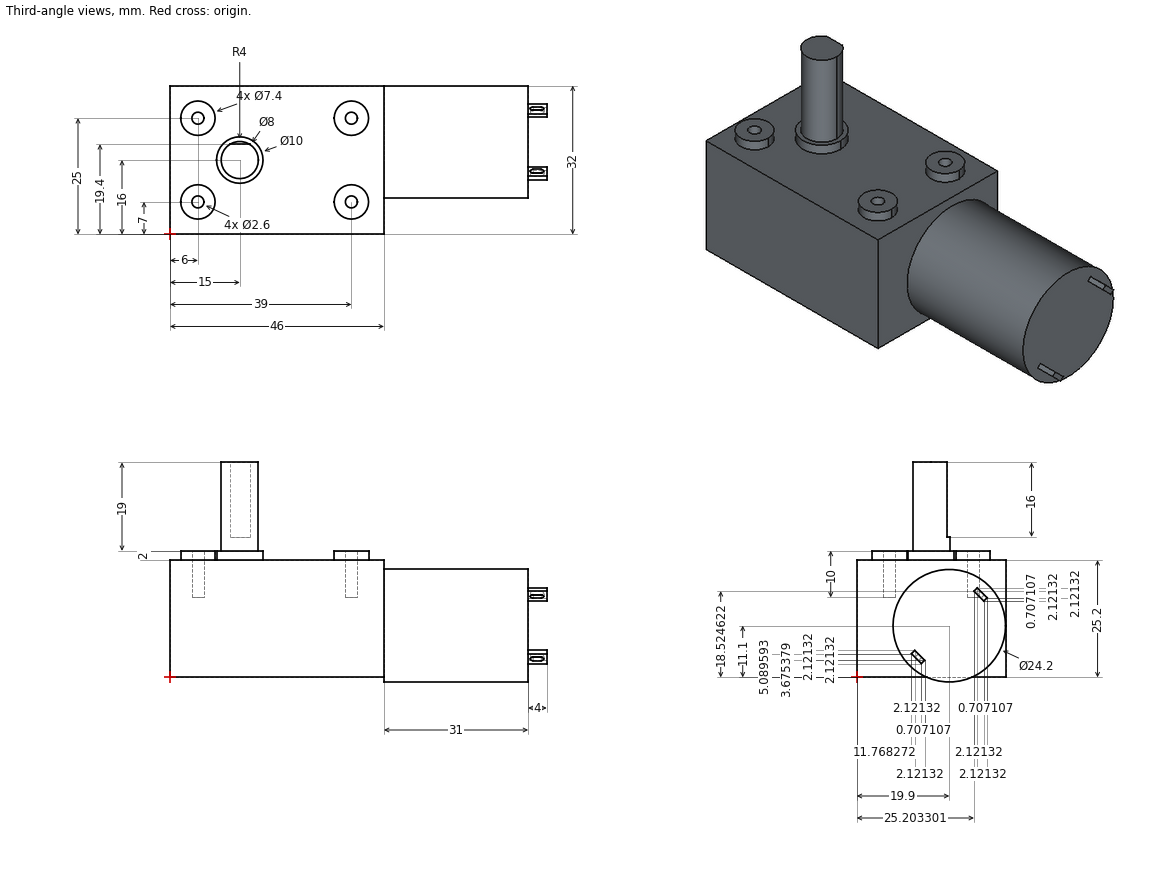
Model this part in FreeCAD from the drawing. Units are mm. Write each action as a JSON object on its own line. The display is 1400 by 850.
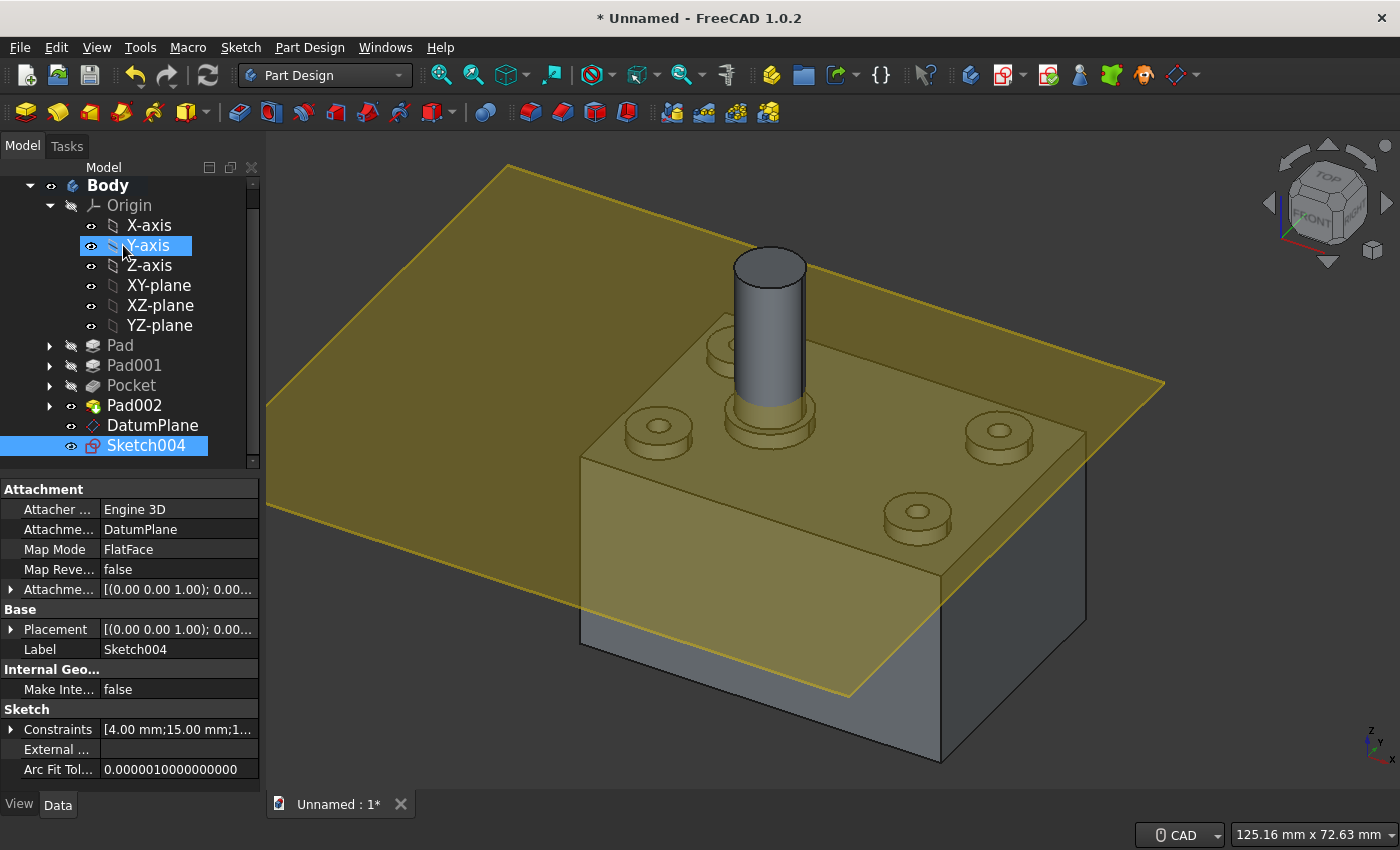
{"action": "left_click", "coordinate": [240, 112]}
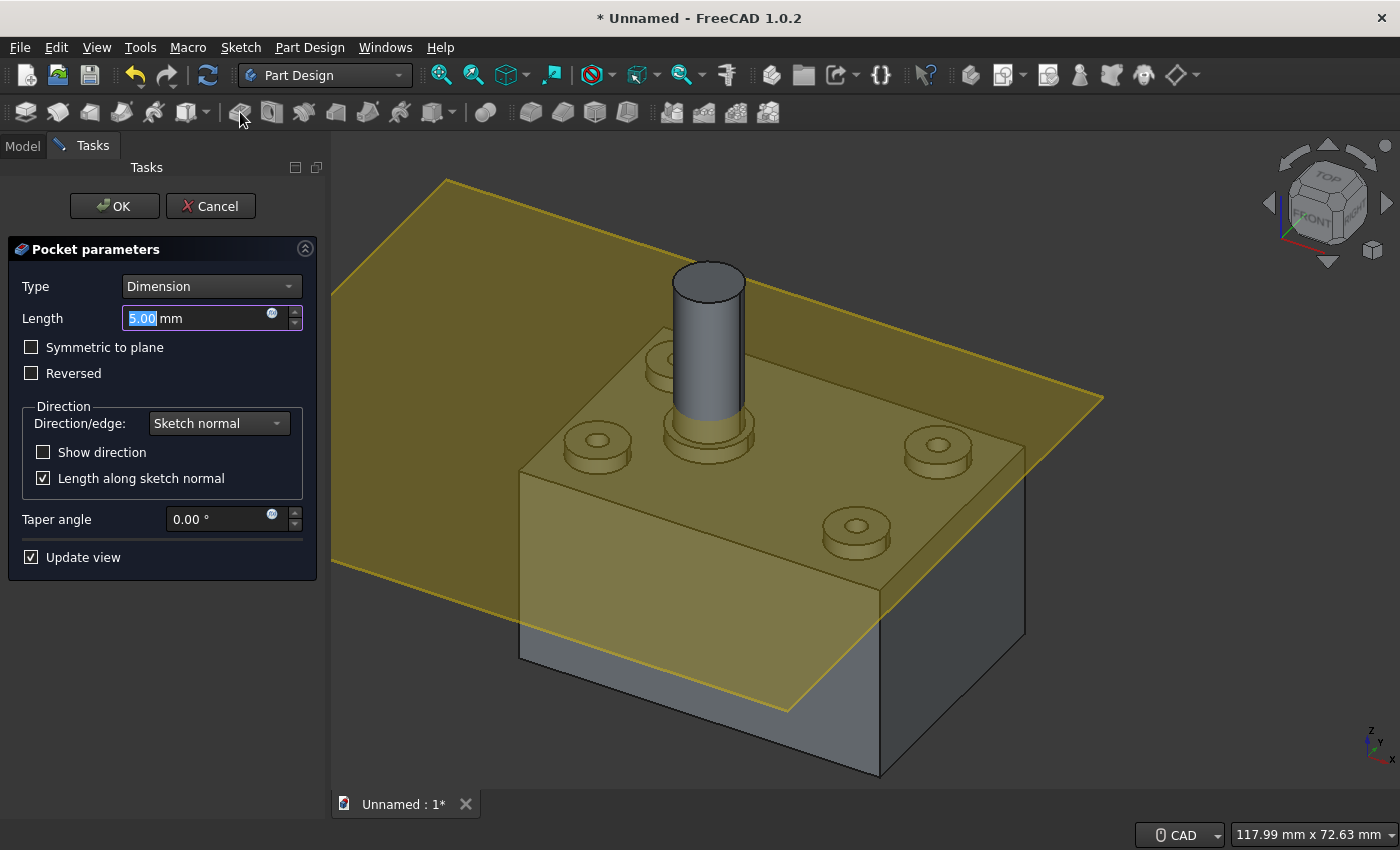
{"action": "type", "text": "16"}
{"action": "key", "text": "Tab"}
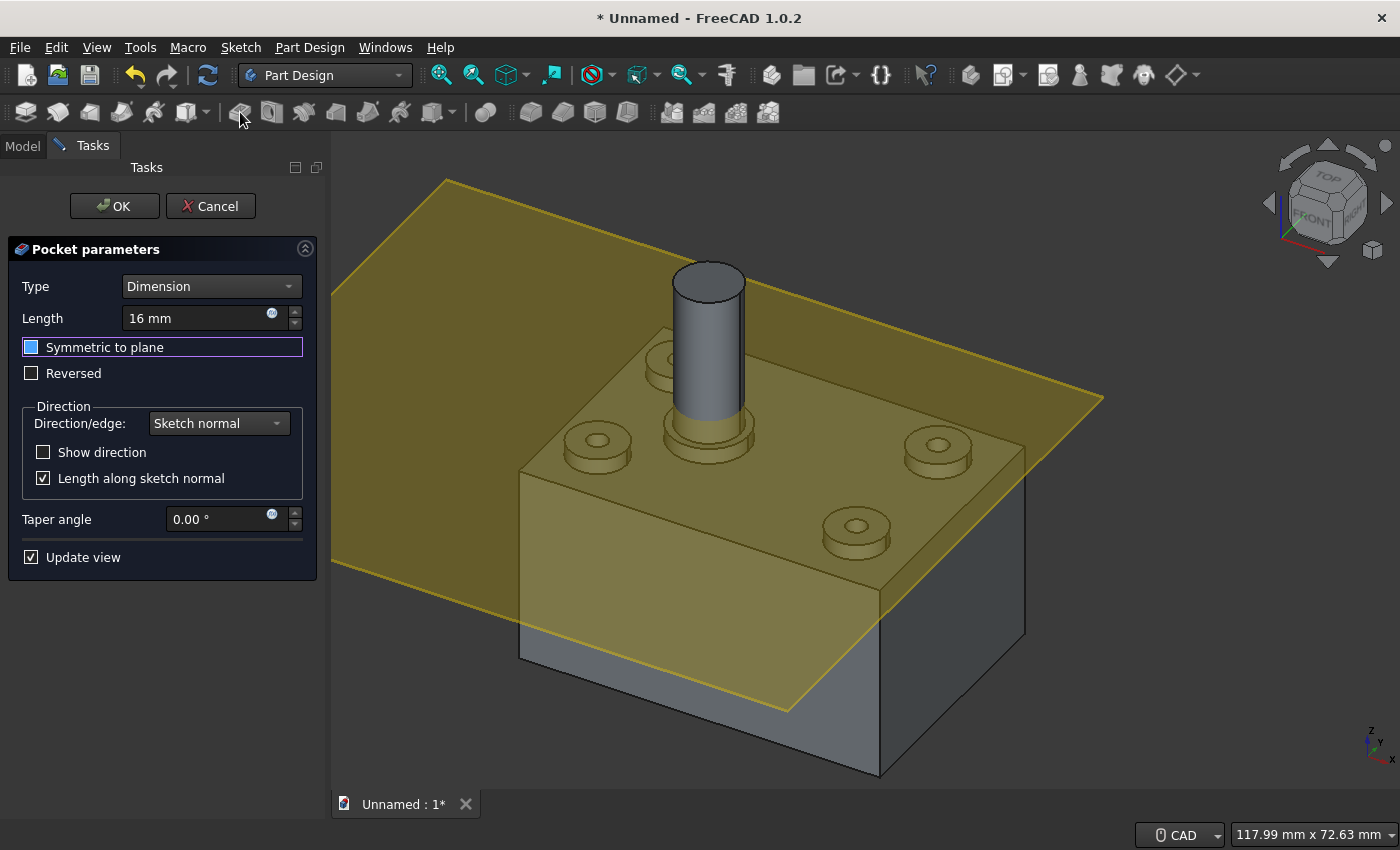
{"action": "left_click", "coordinate": [30, 373]}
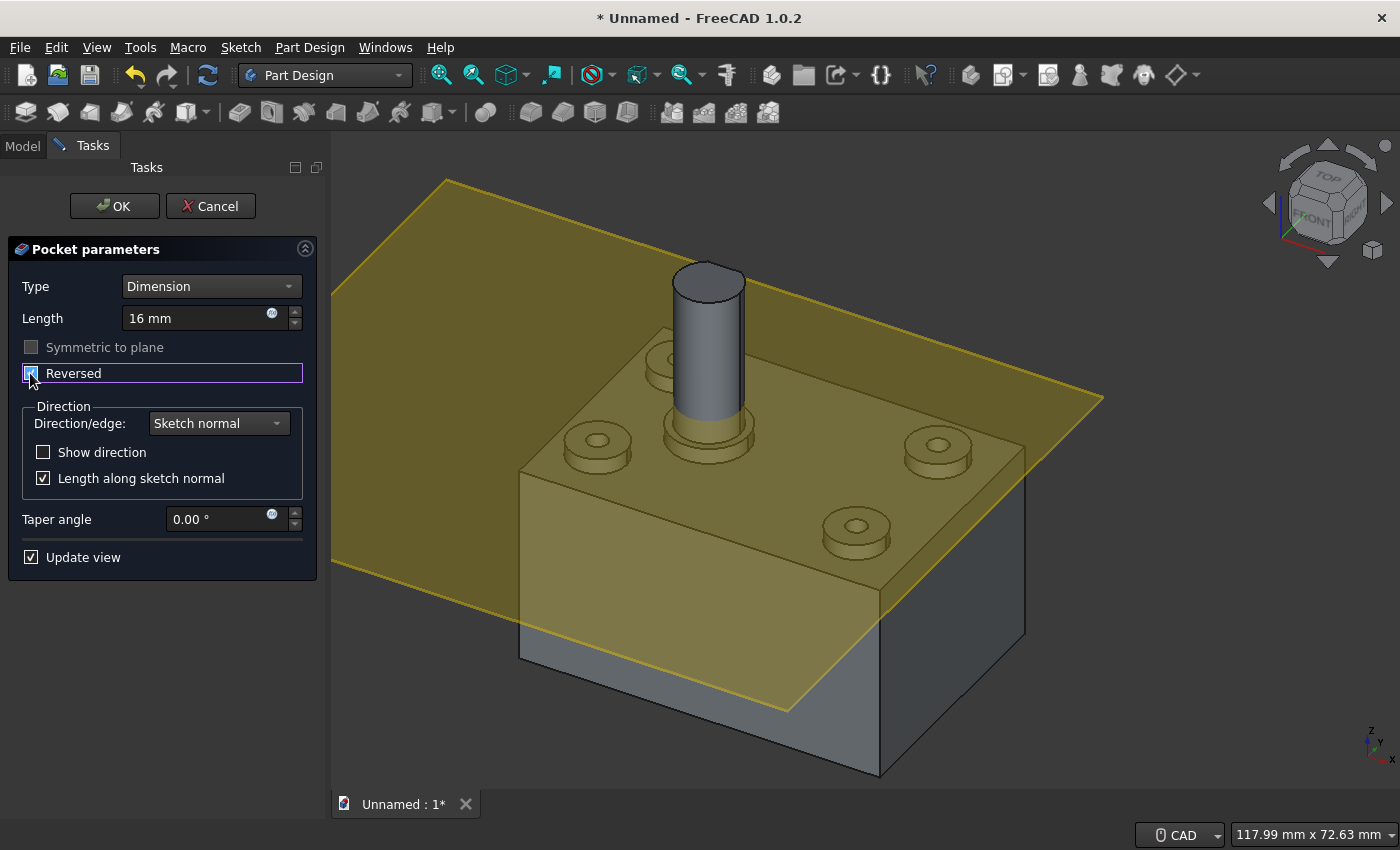
{"action": "left_click", "coordinate": [115, 206]}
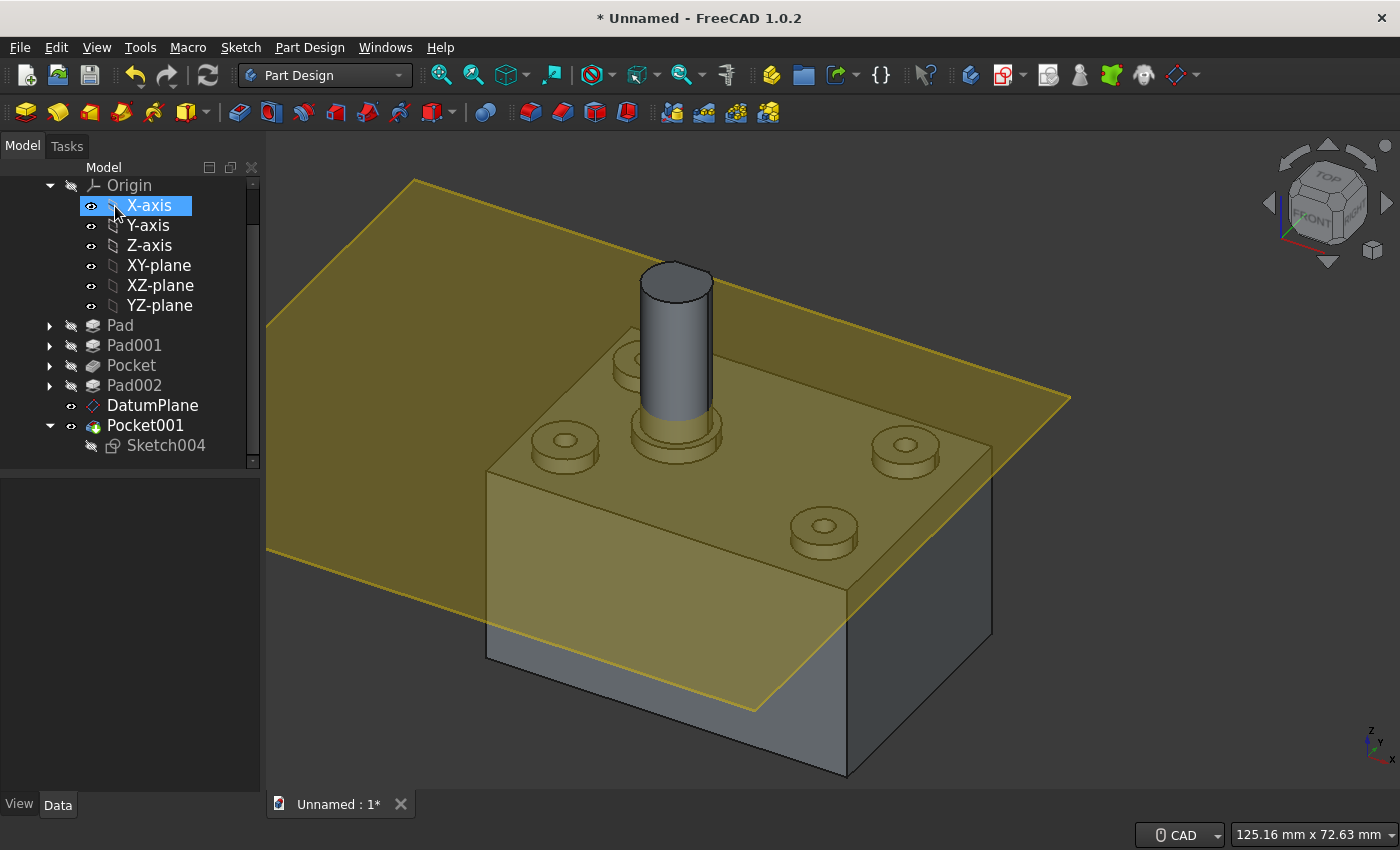
{"action": "left_click", "coordinate": [116, 406]}
{"action": "key", "text": "space"}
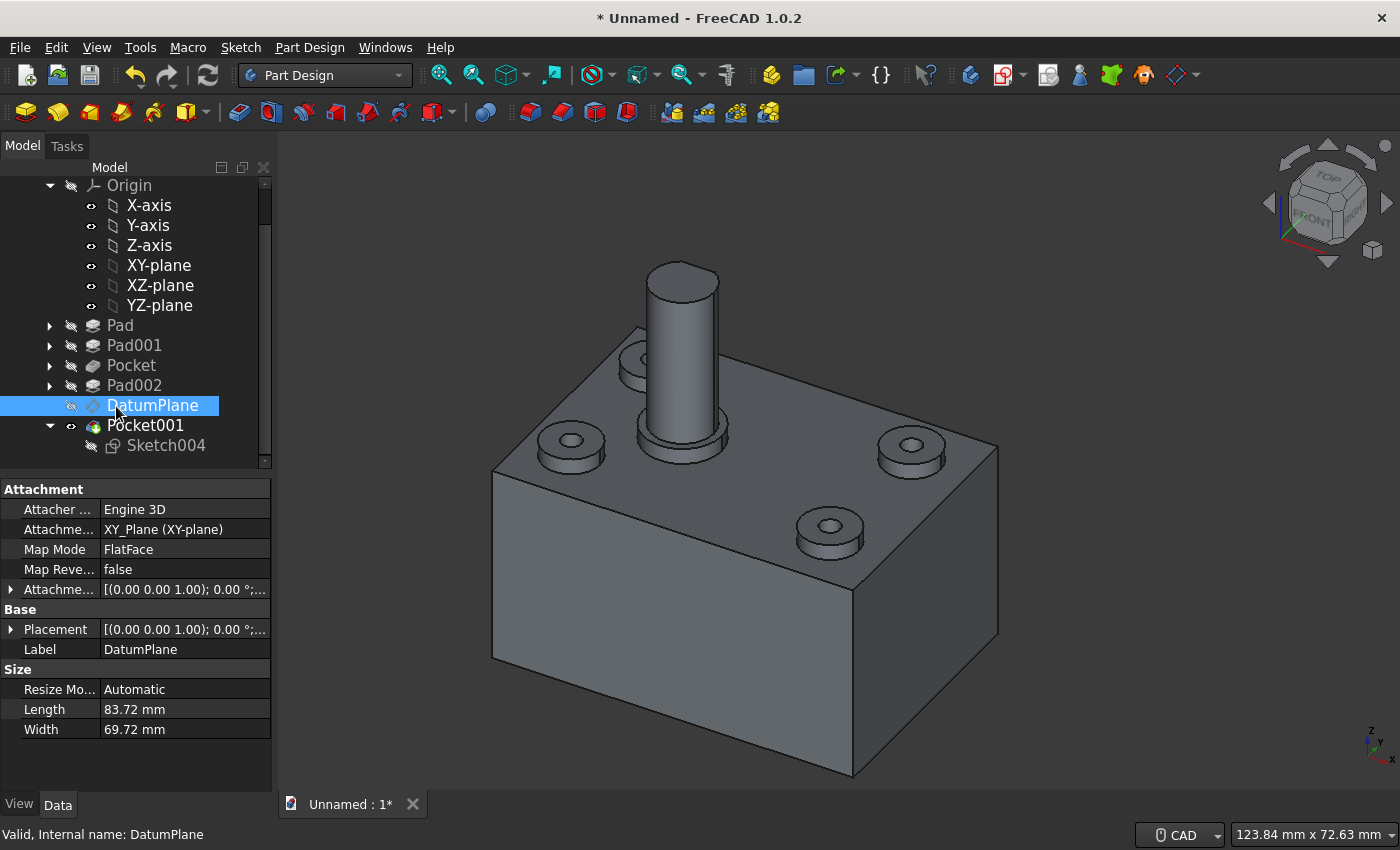
{"action": "left_click", "coordinate": [926, 611]}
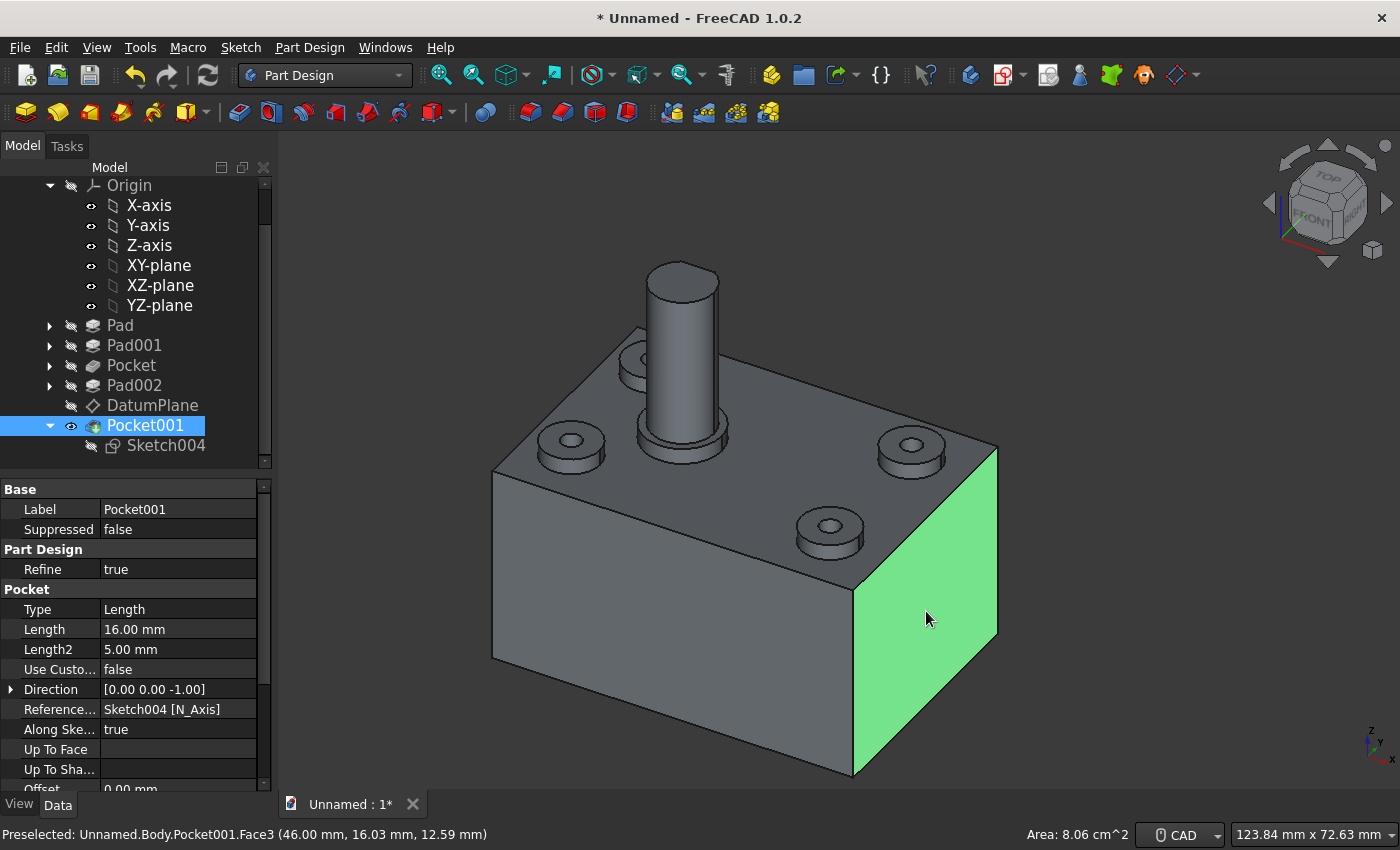
{"action": "left_click", "coordinate": [1004, 76]}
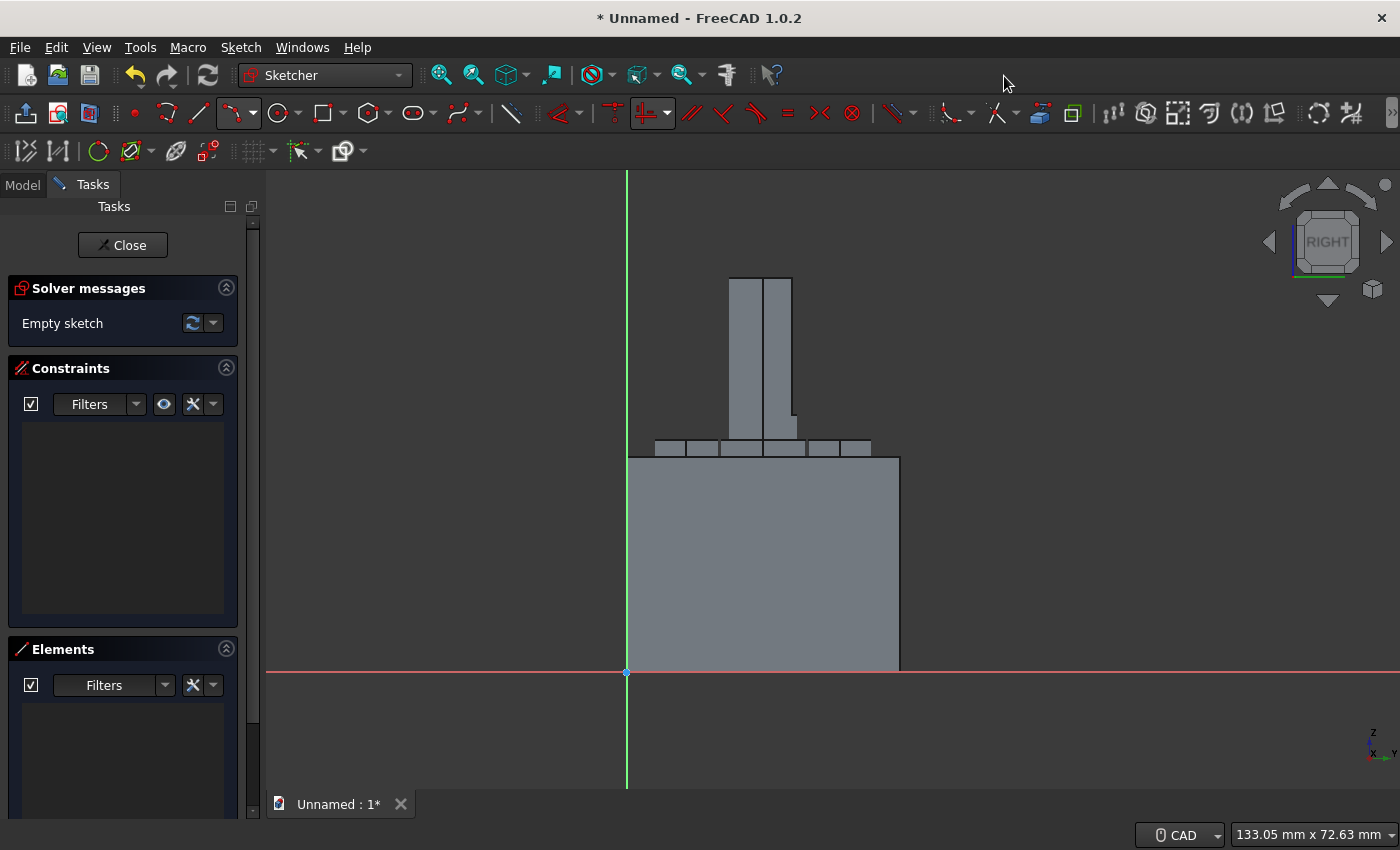
{"action": "scroll", "coordinate": [762, 697], "scroll_direction": "up", "scroll_amount": 3}